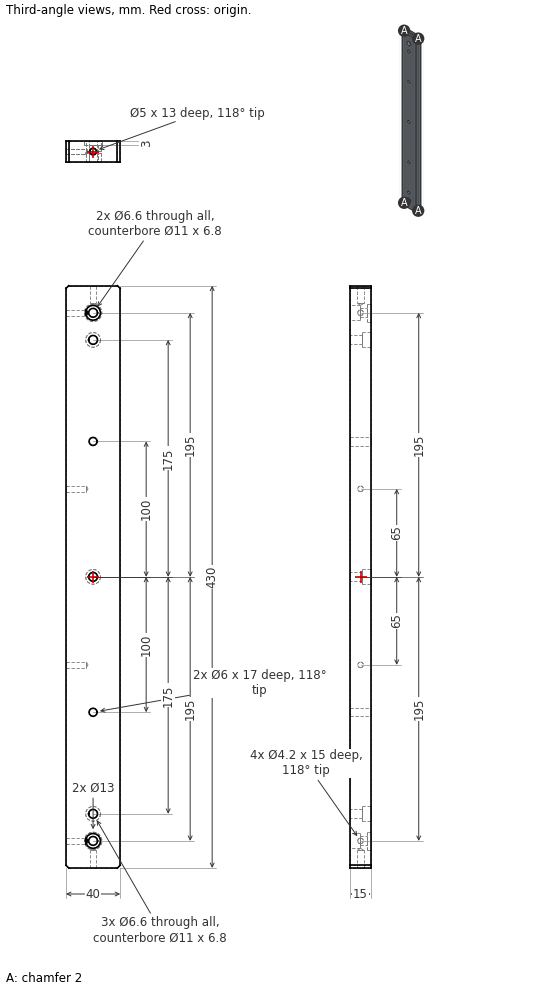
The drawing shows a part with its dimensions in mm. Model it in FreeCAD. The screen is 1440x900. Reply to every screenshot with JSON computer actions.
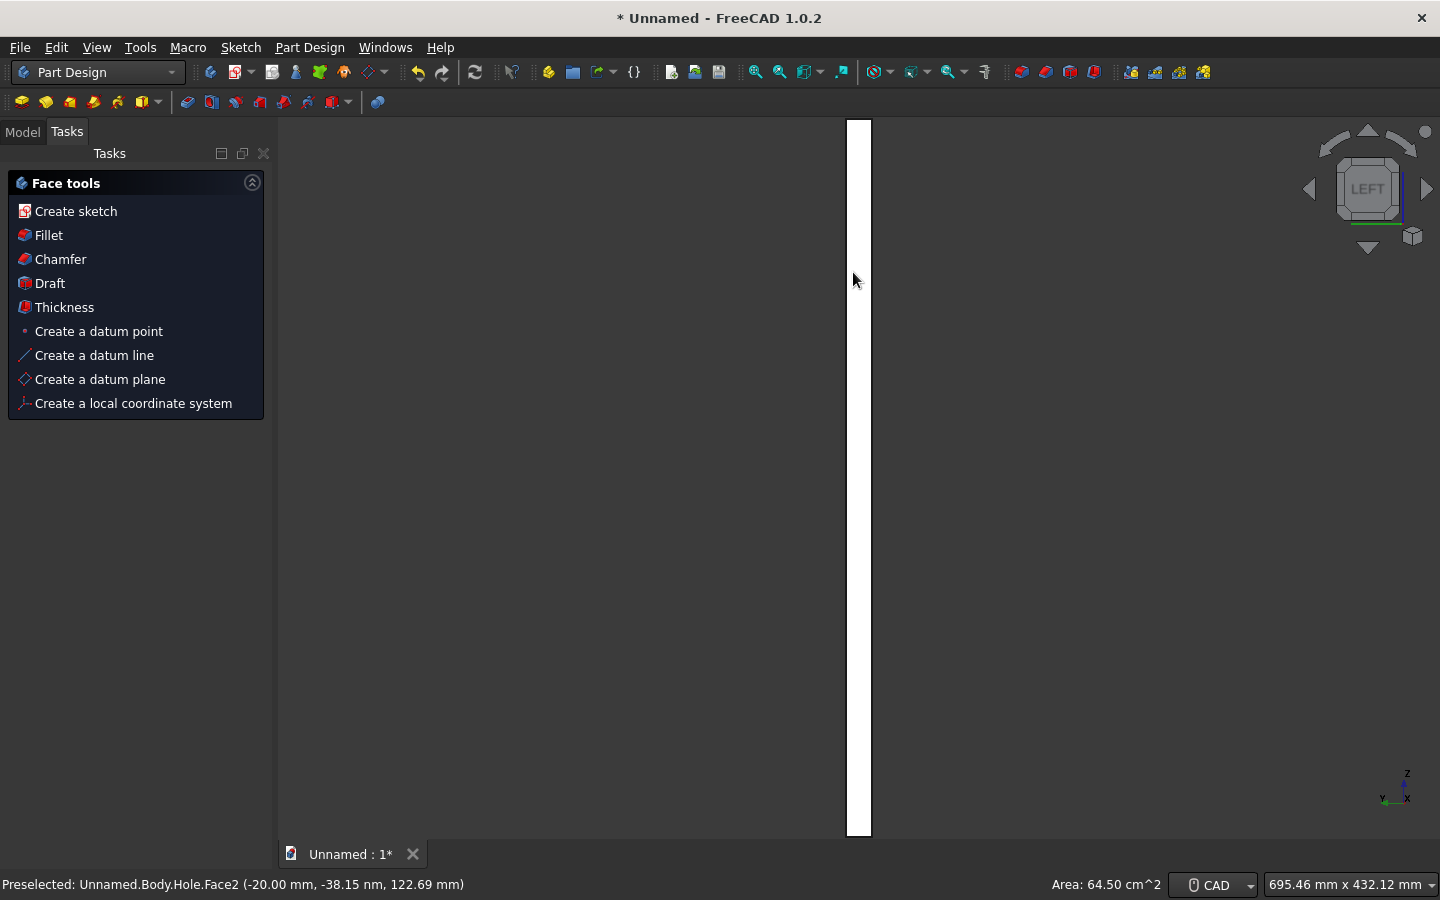
{"action": "left_click", "coordinate": [236, 72]}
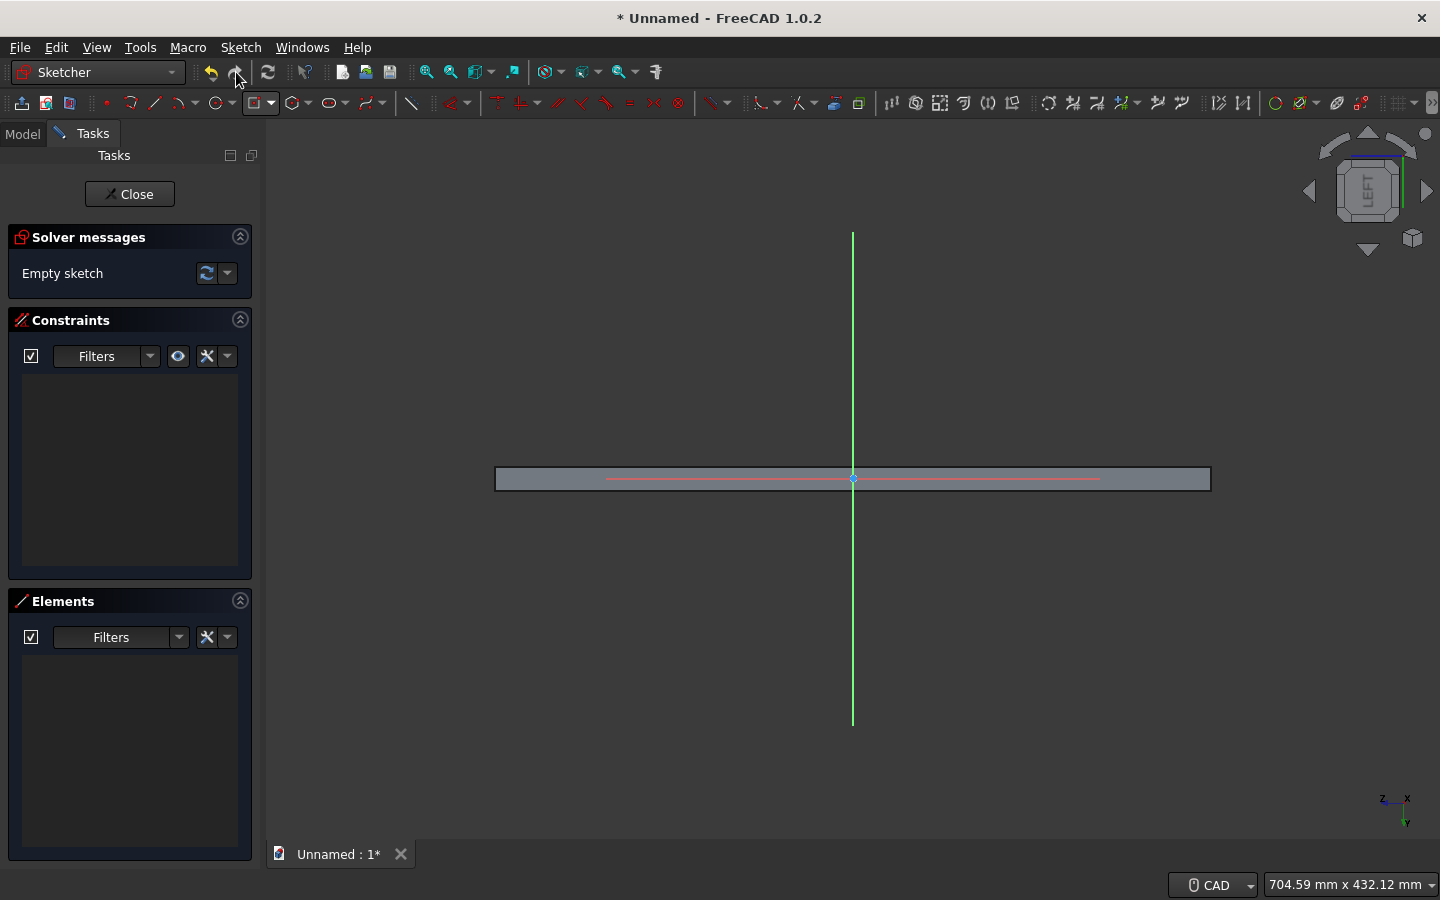
{"action": "left_click", "coordinate": [216, 104]}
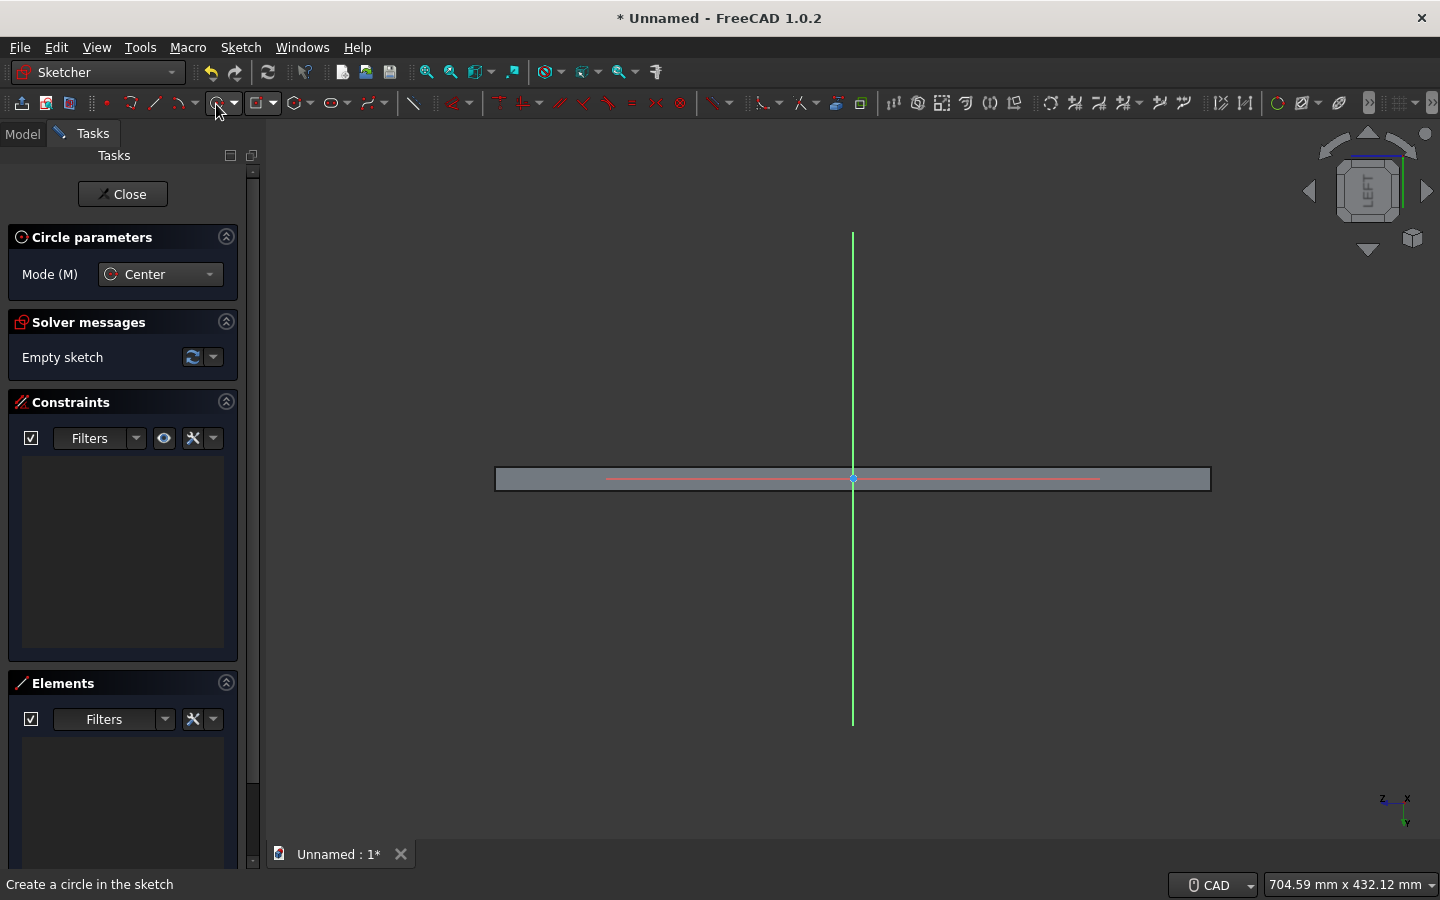
{"action": "scroll", "coordinate": [1178, 479], "scroll_direction": "up", "scroll_amount": 10}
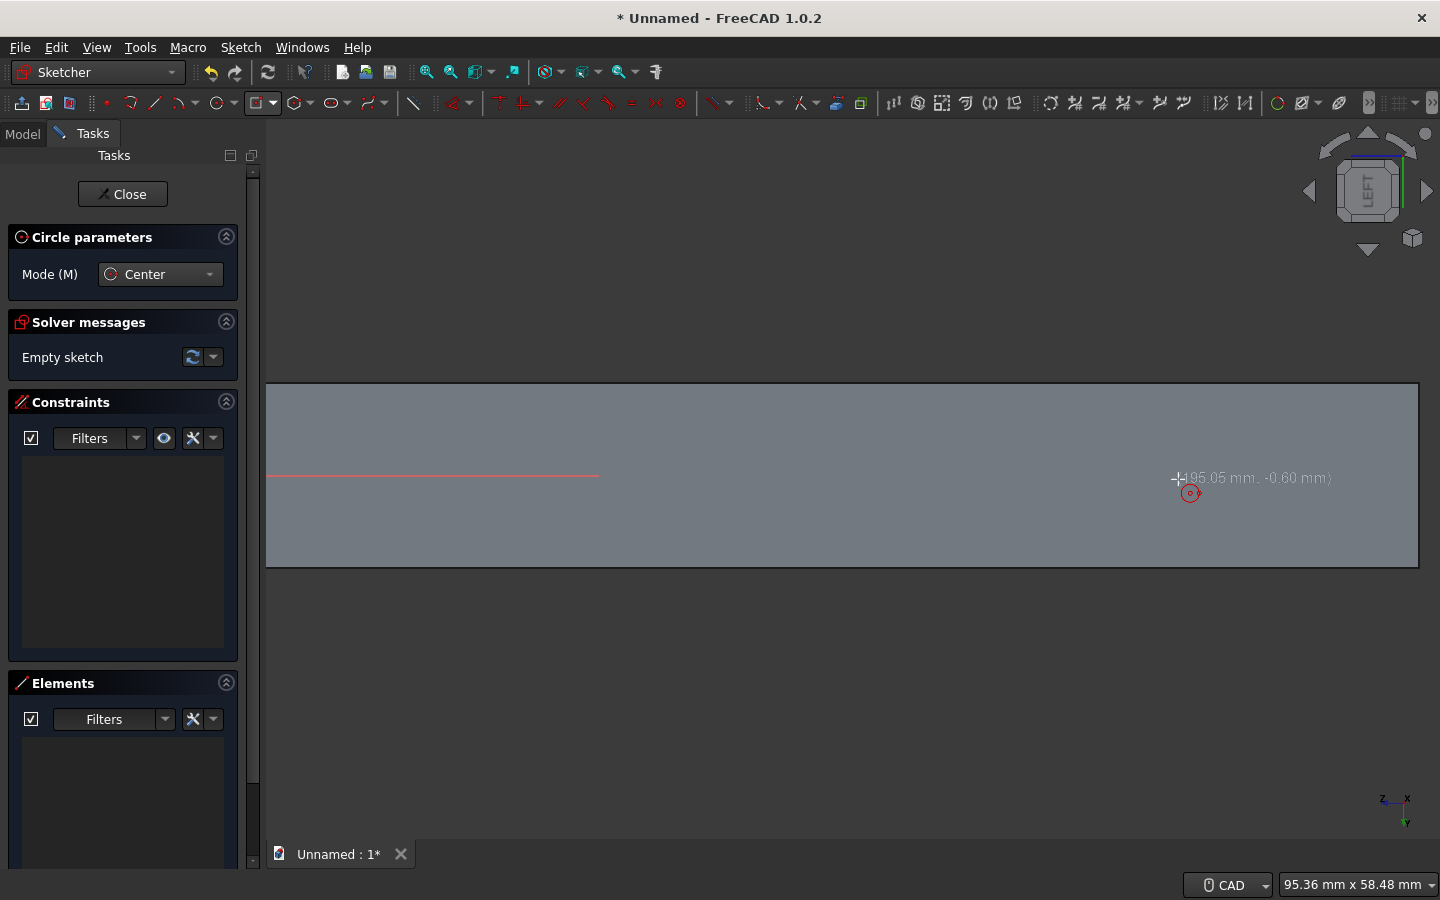
{"action": "scroll", "coordinate": [1100, 480], "scroll_direction": "down", "scroll_amount": 10}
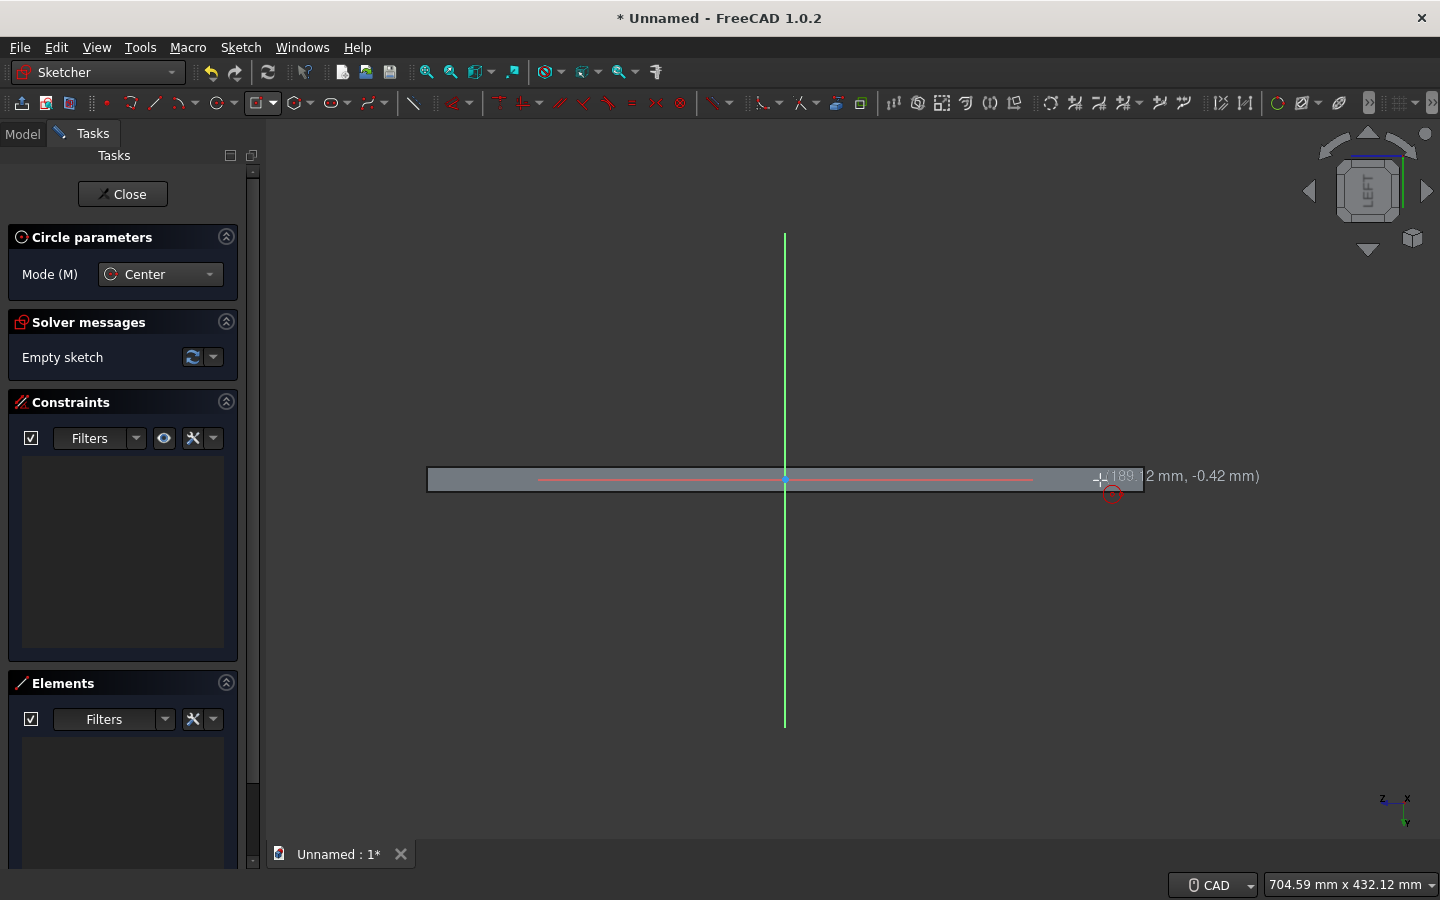
{"action": "left_click", "coordinate": [1110, 480]}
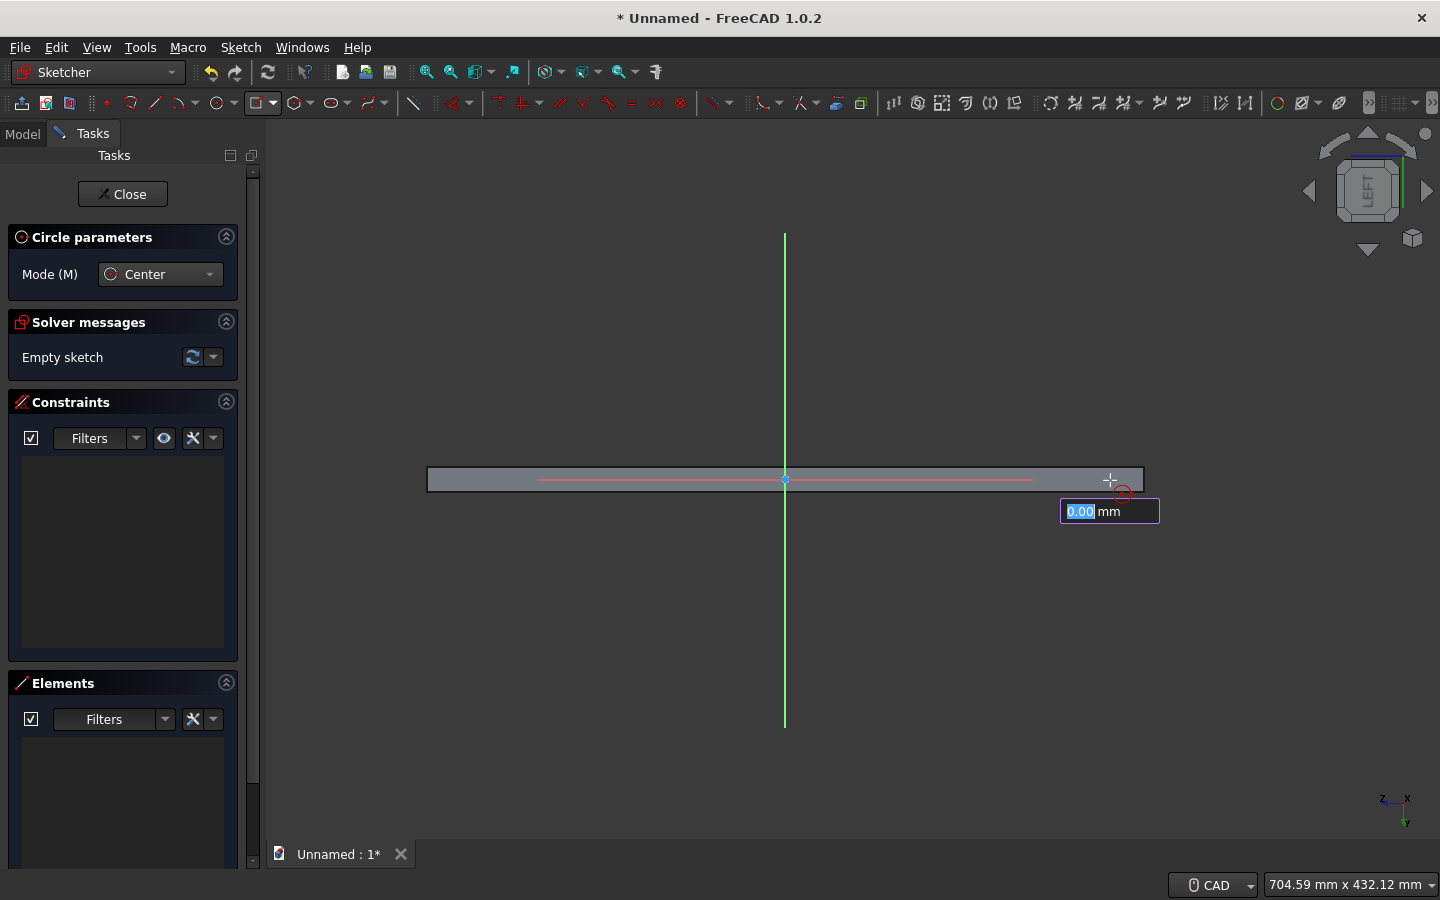
{"action": "scroll", "coordinate": [1109, 483], "scroll_direction": "up", "scroll_amount": 8}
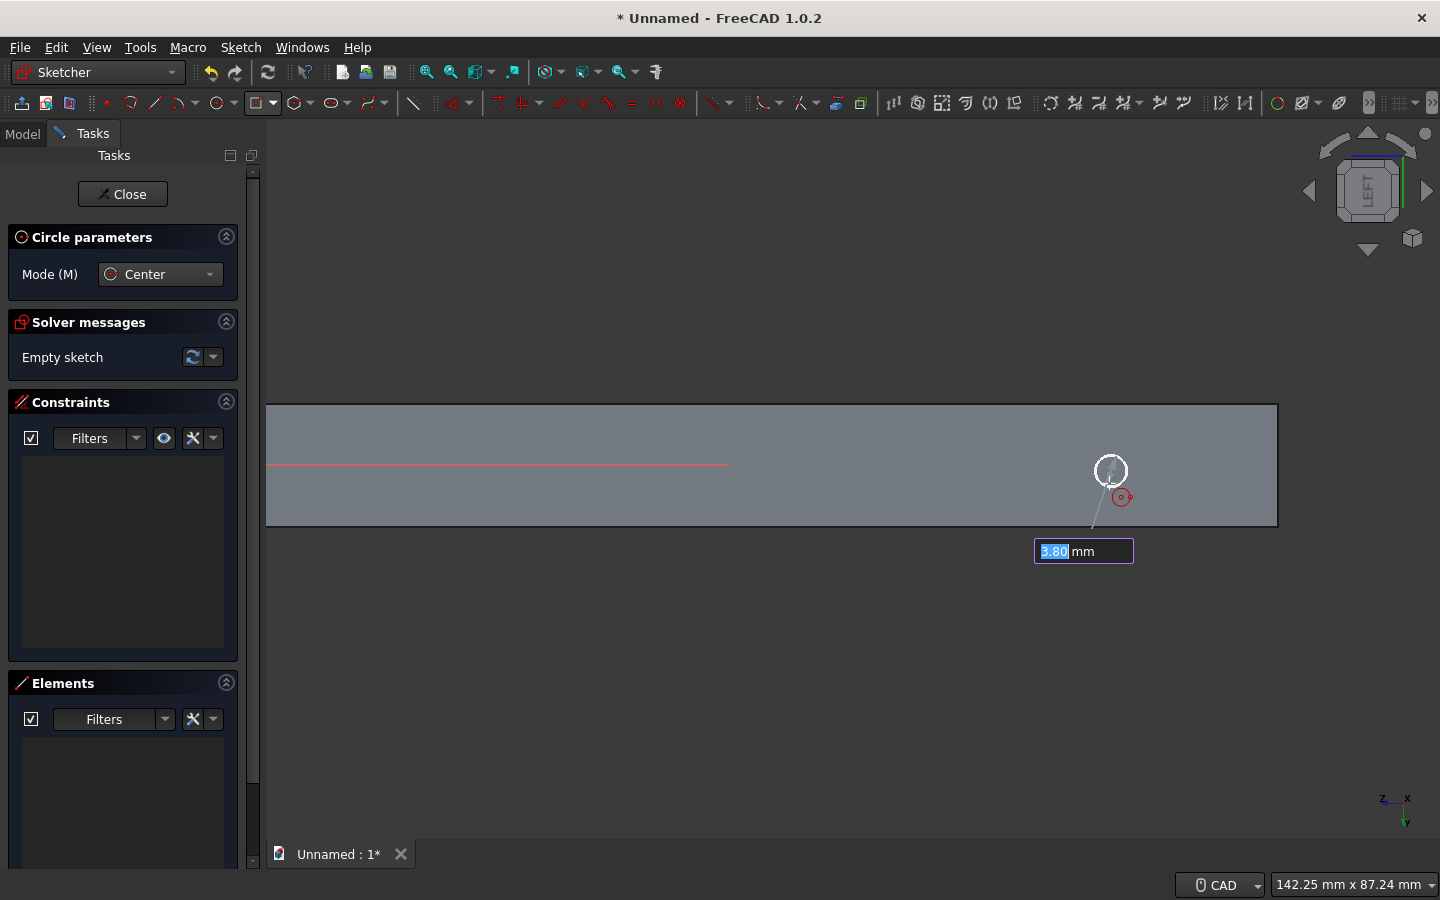
{"action": "left_click", "coordinate": [1107, 482]}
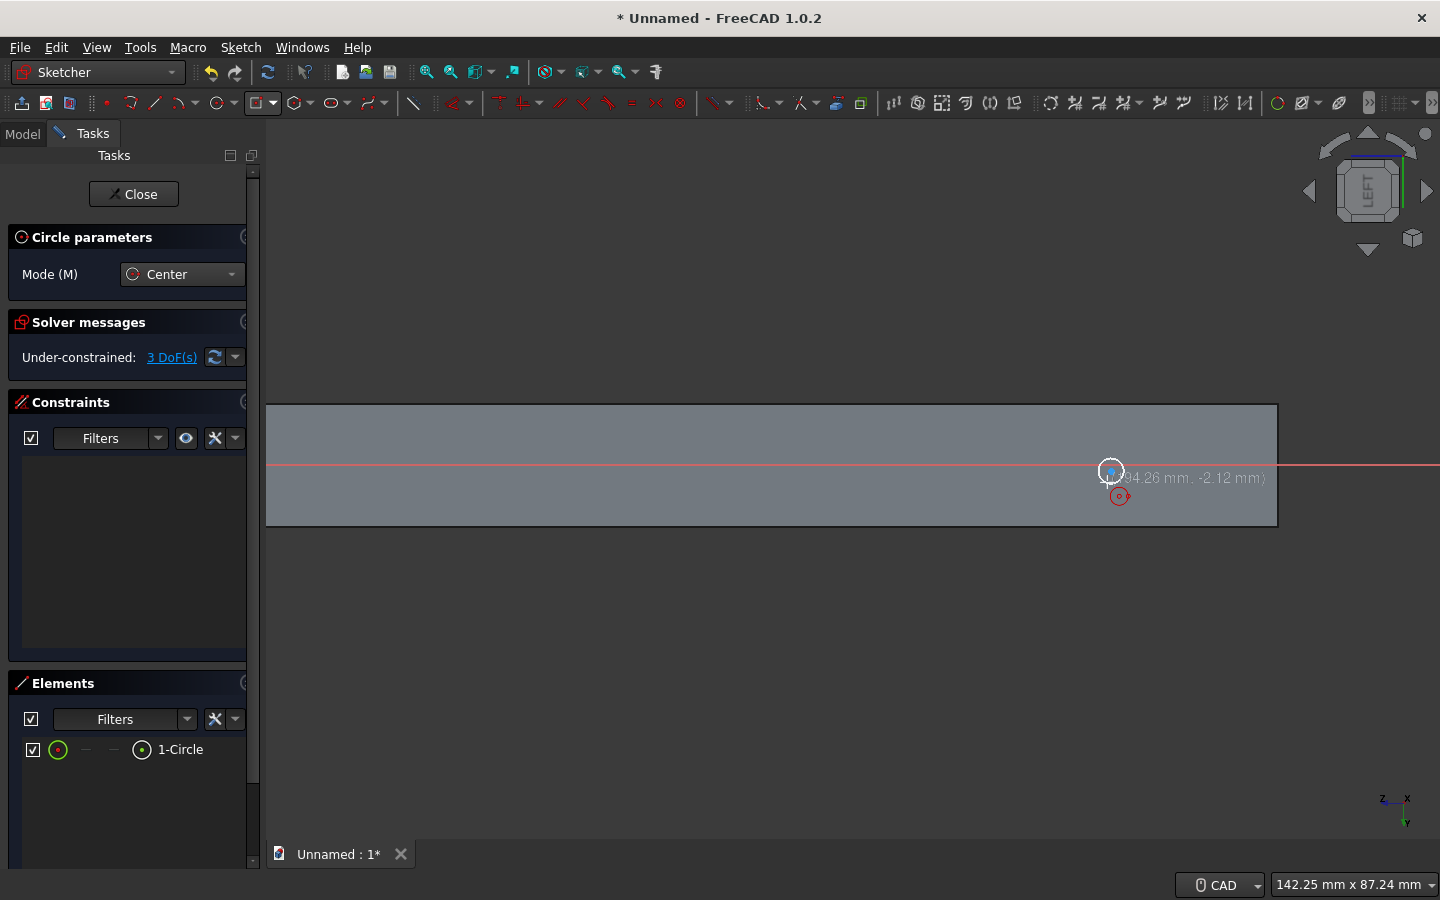
{"action": "scroll", "coordinate": [1108, 482], "scroll_direction": "down", "scroll_amount": 8}